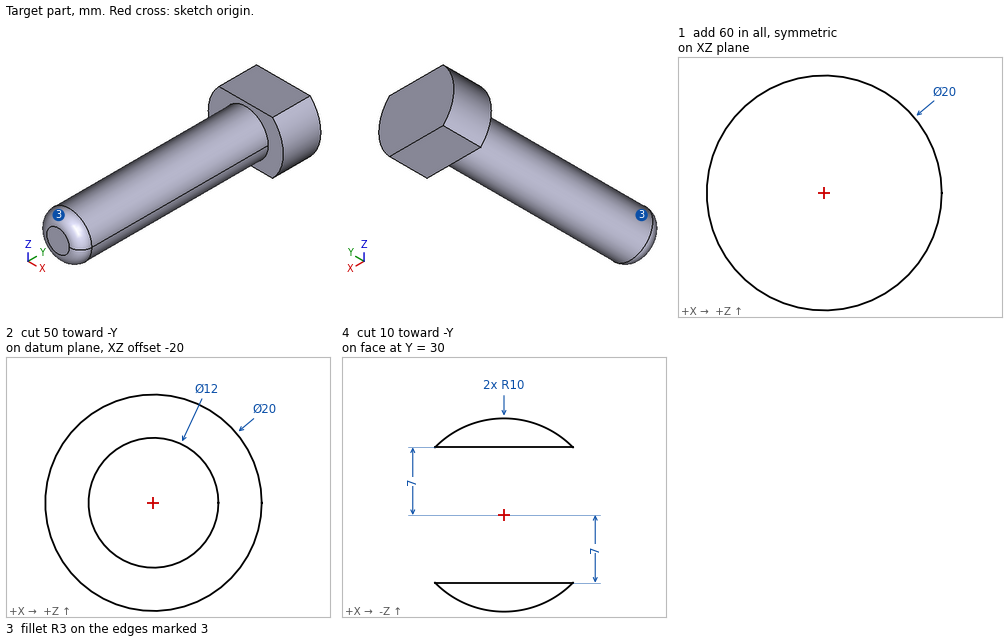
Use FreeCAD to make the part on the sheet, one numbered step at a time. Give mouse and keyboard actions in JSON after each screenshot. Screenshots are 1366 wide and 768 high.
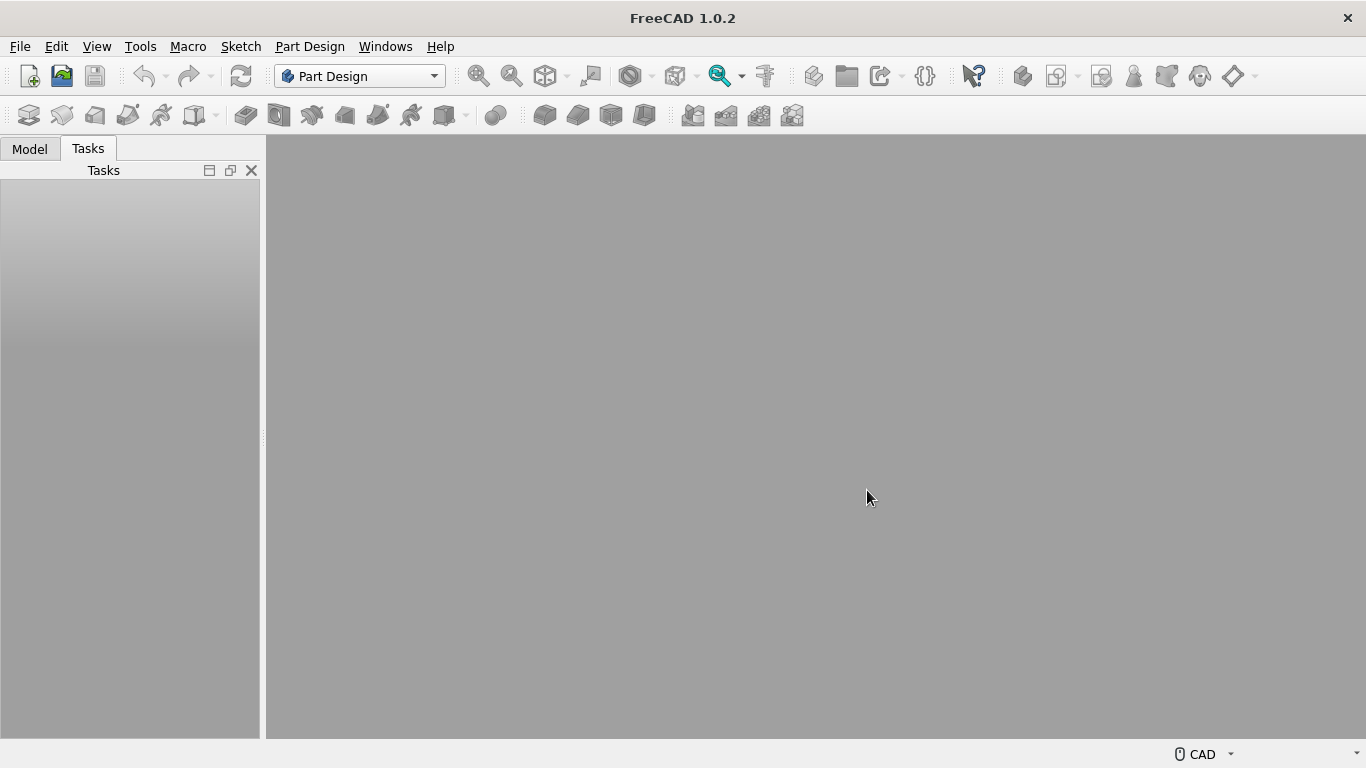
{"action": "left_click", "coordinate": [29, 76]}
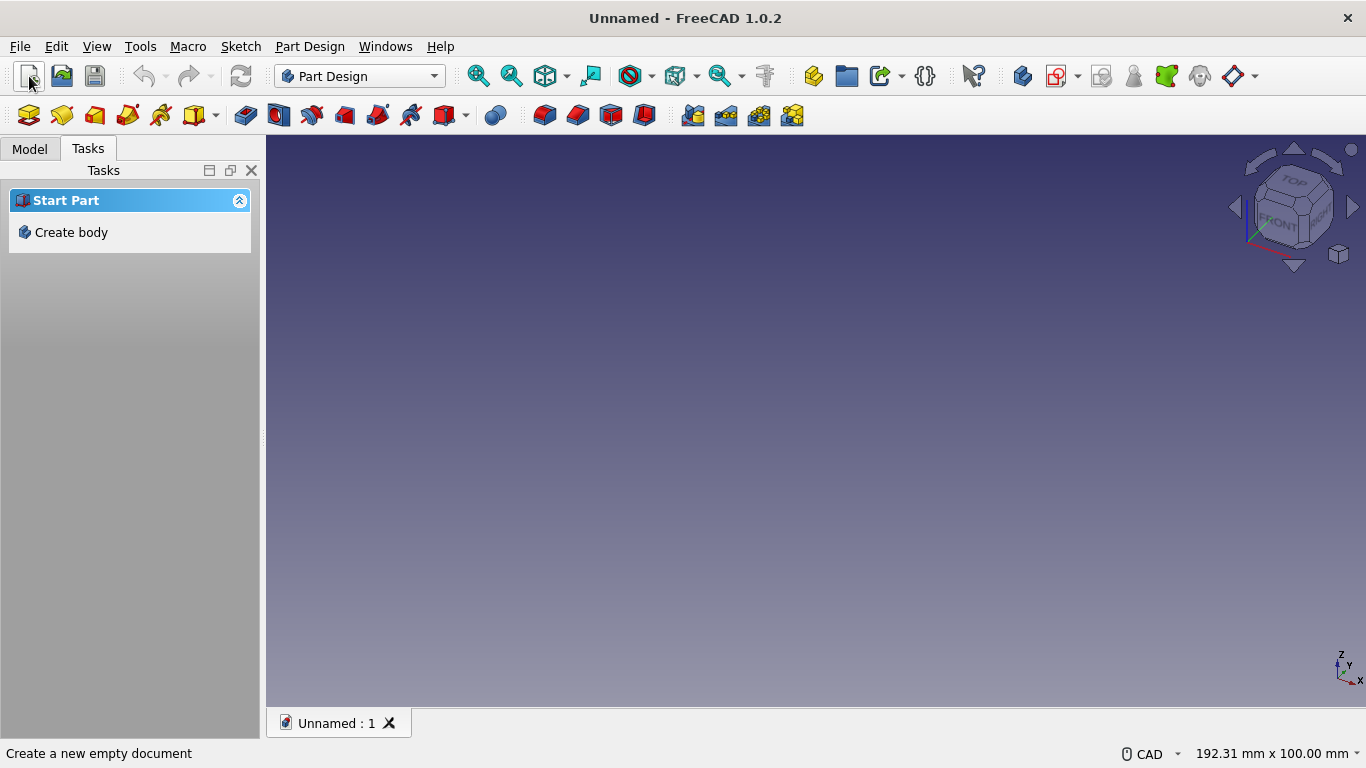
{"action": "left_click", "coordinate": [1056, 76]}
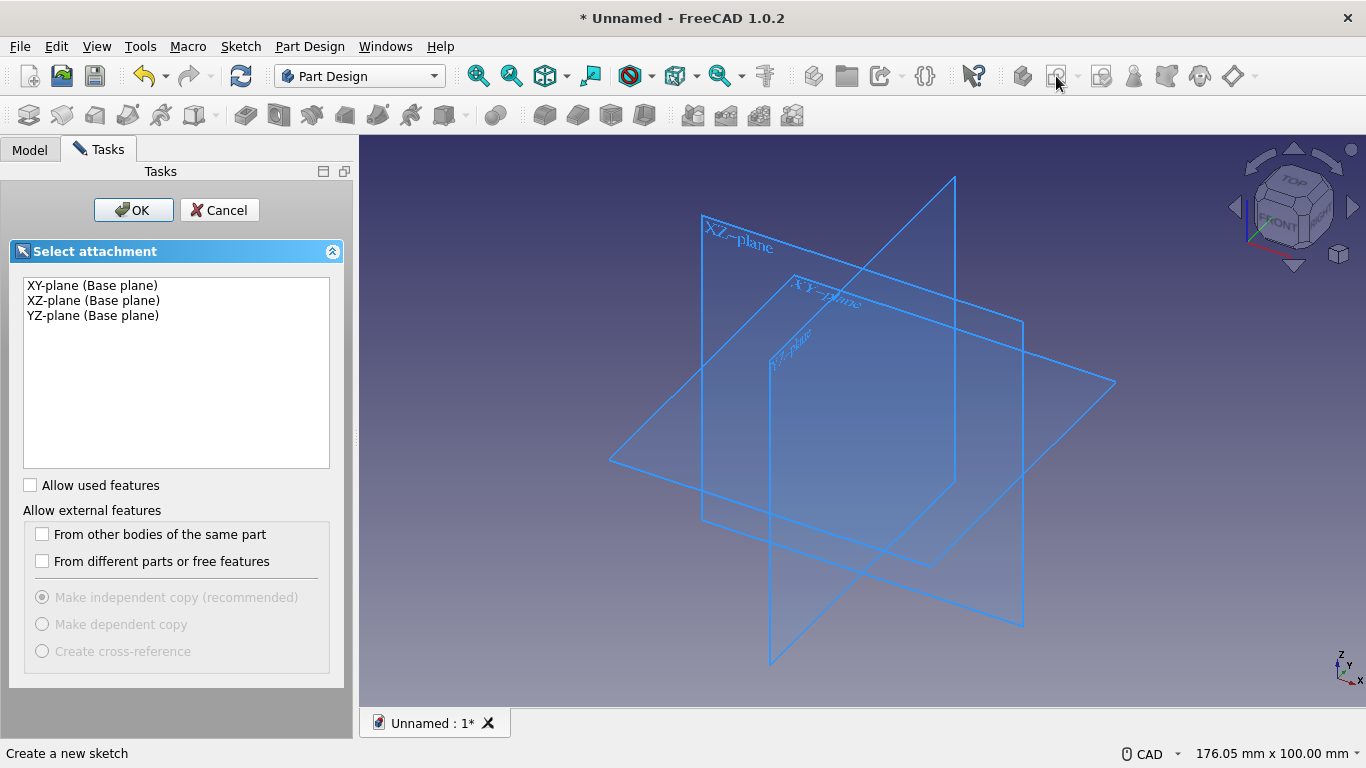
{"action": "left_click", "coordinate": [84, 300]}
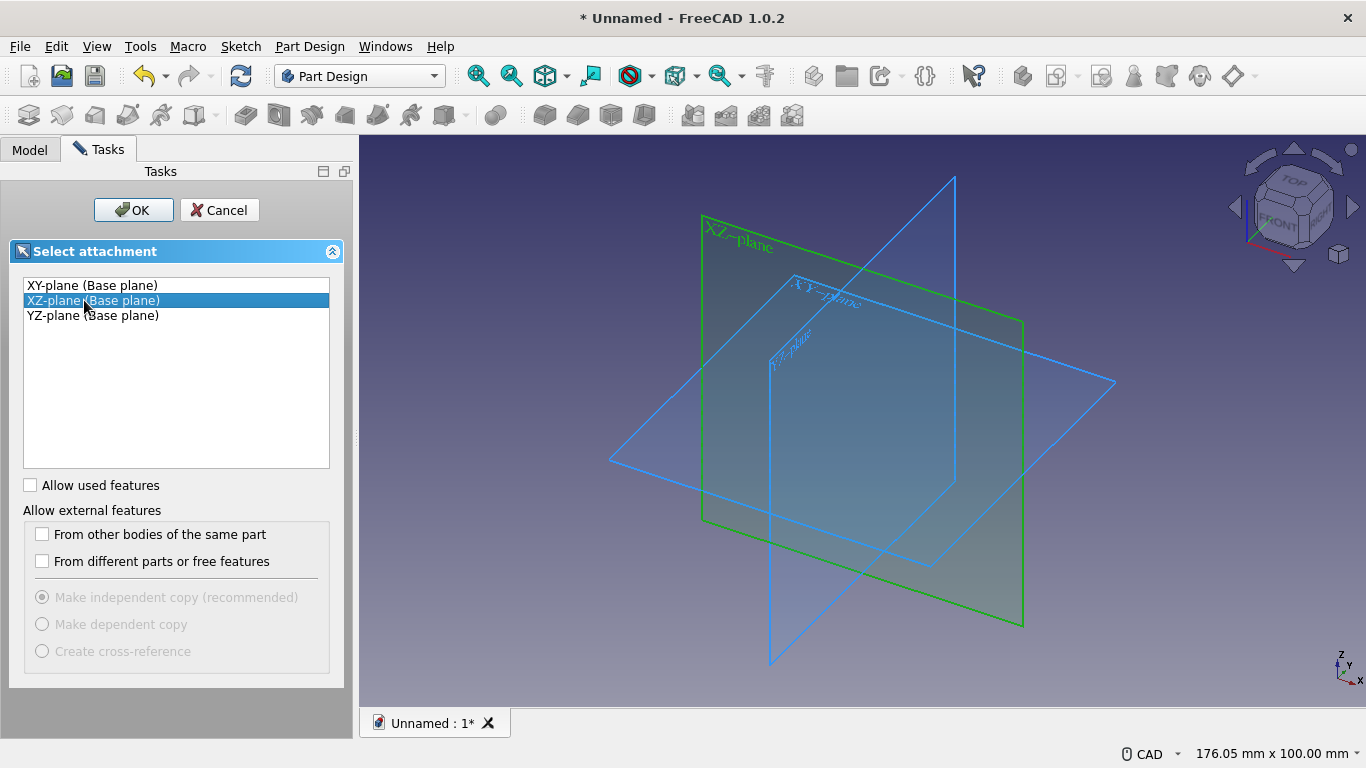
{"action": "left_click", "coordinate": [134, 210]}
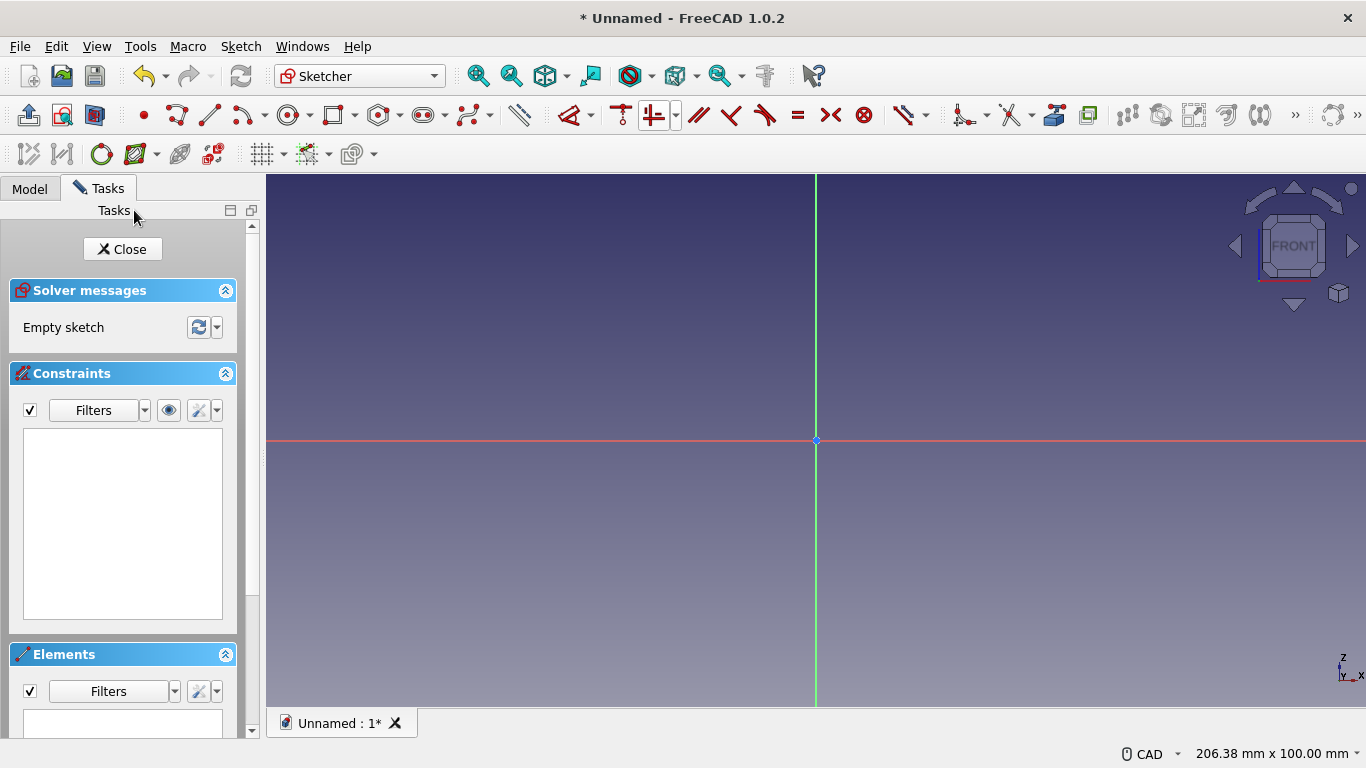
{"action": "scroll", "coordinate": [846, 440], "scroll_direction": "up", "scroll_amount": 6}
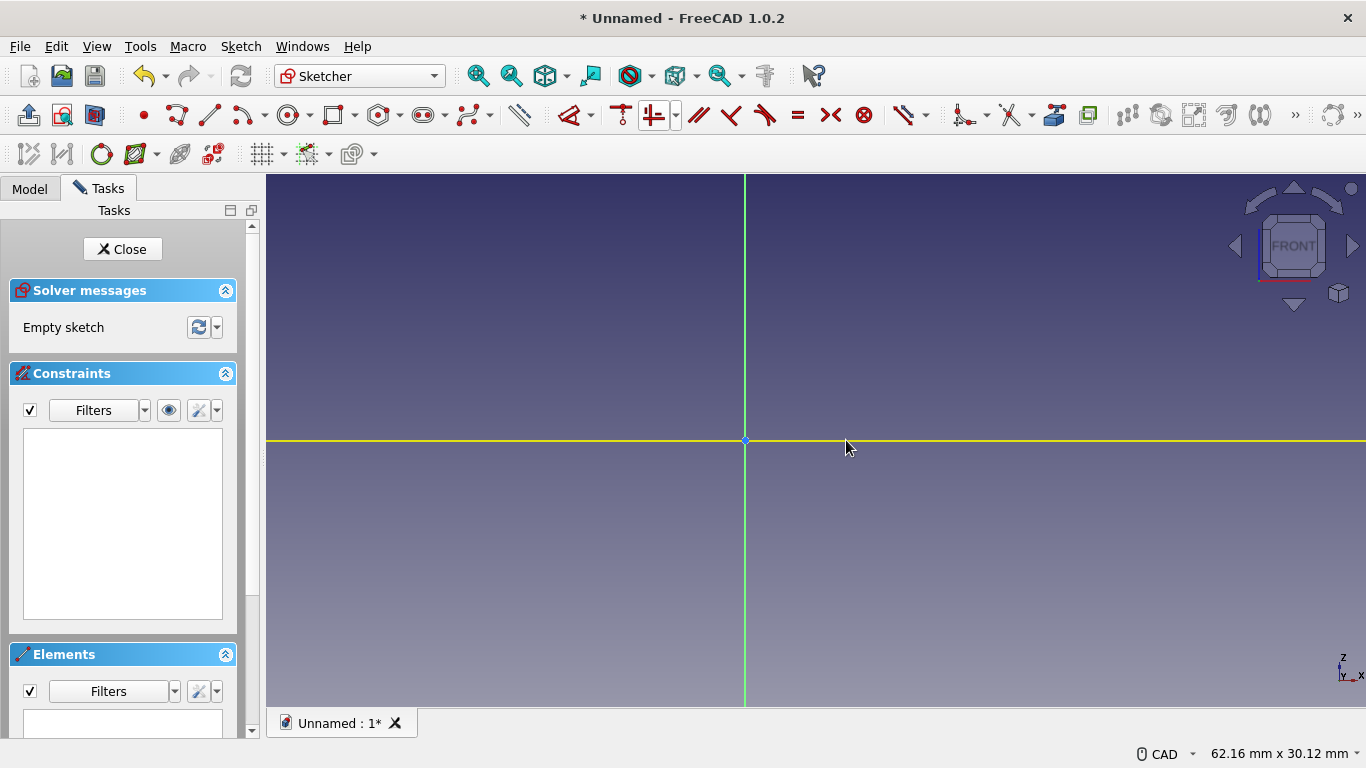
{"action": "left_click", "coordinate": [288, 116]}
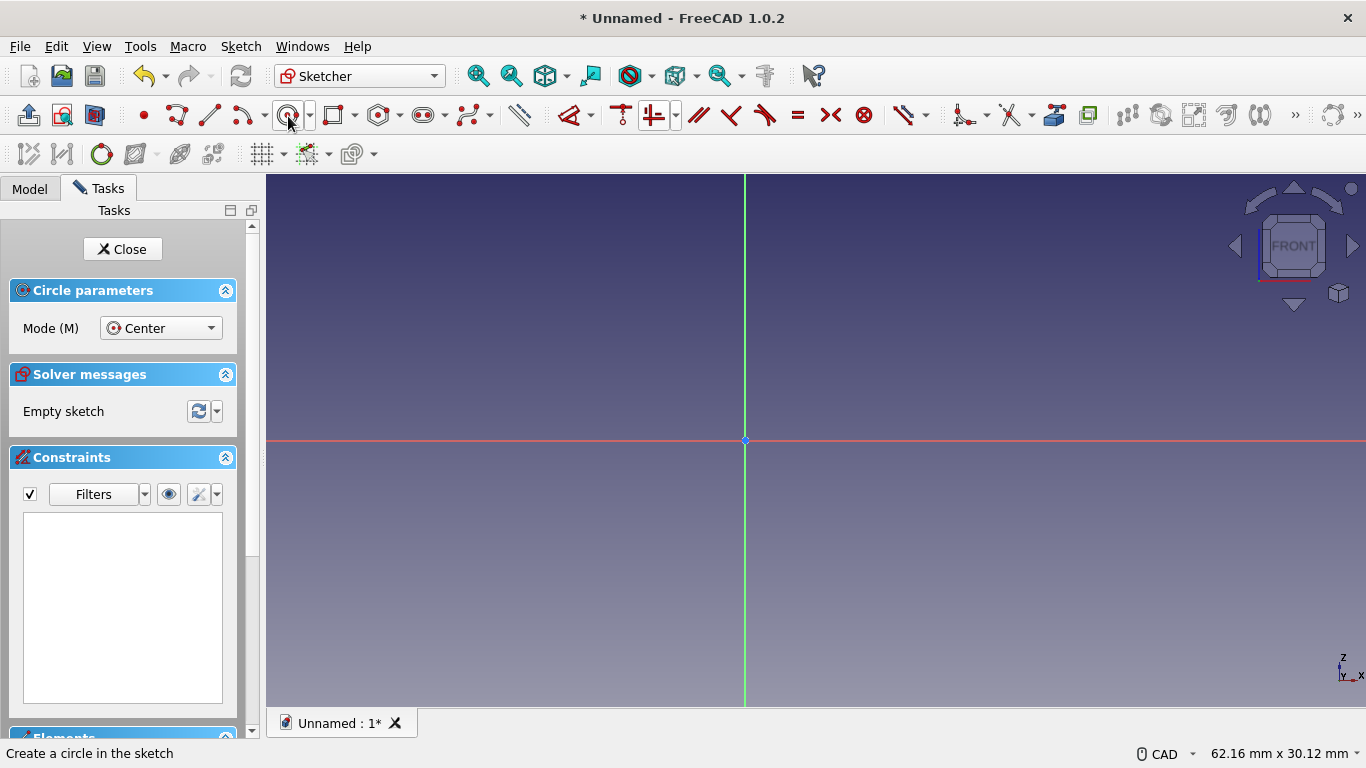
{"action": "left_click", "coordinate": [745, 440]}
{"action": "mouse_move", "coordinate": [870, 315]}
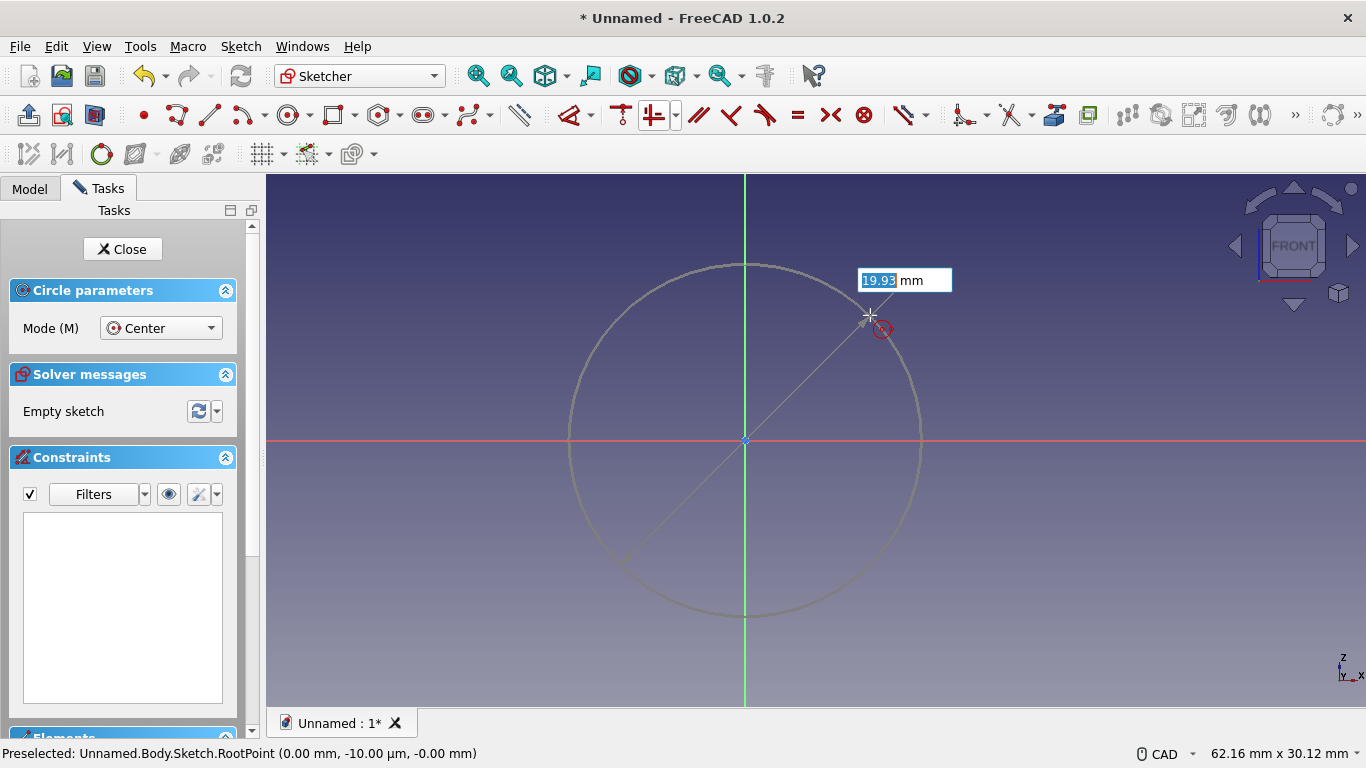
{"action": "type", "text": "20"}
{"action": "key", "text": "Return"}
{"action": "key", "text": "Escape"}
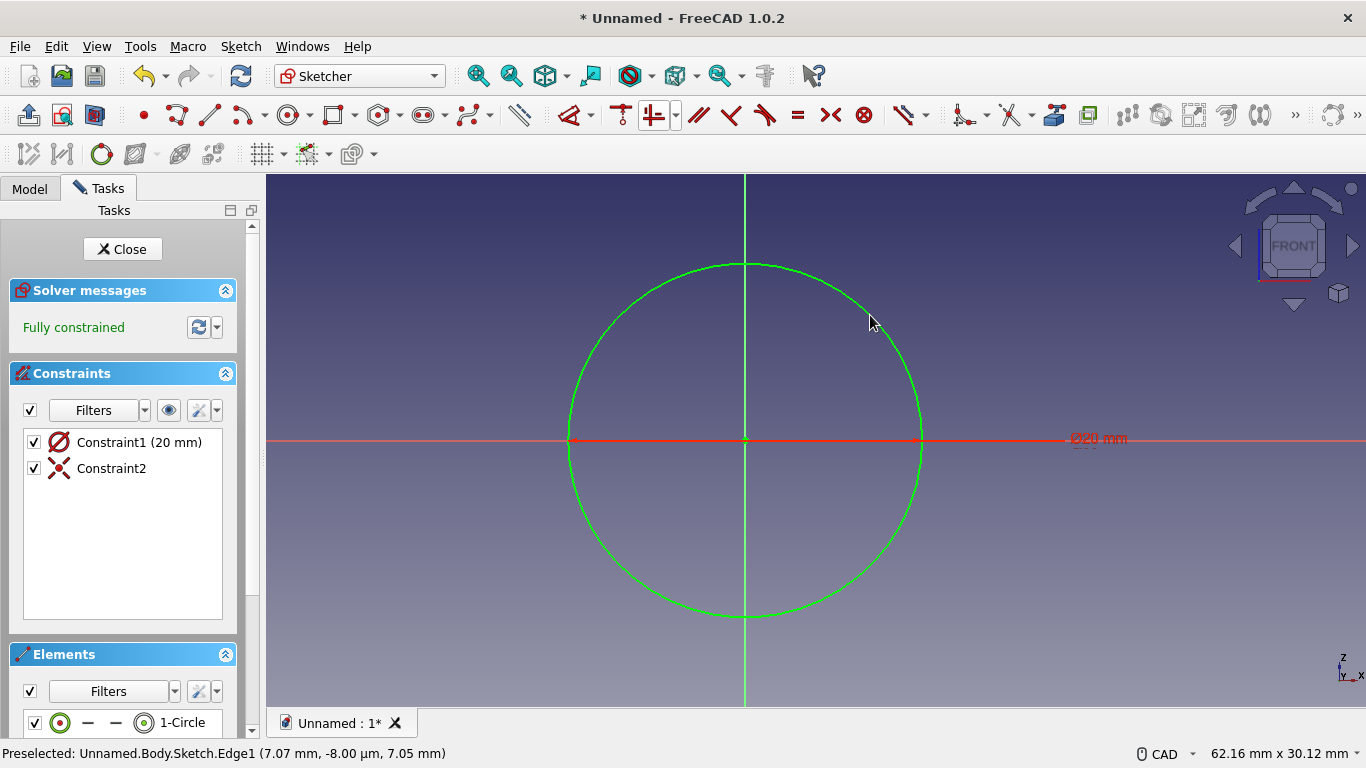
{"action": "left_click", "coordinate": [123, 249]}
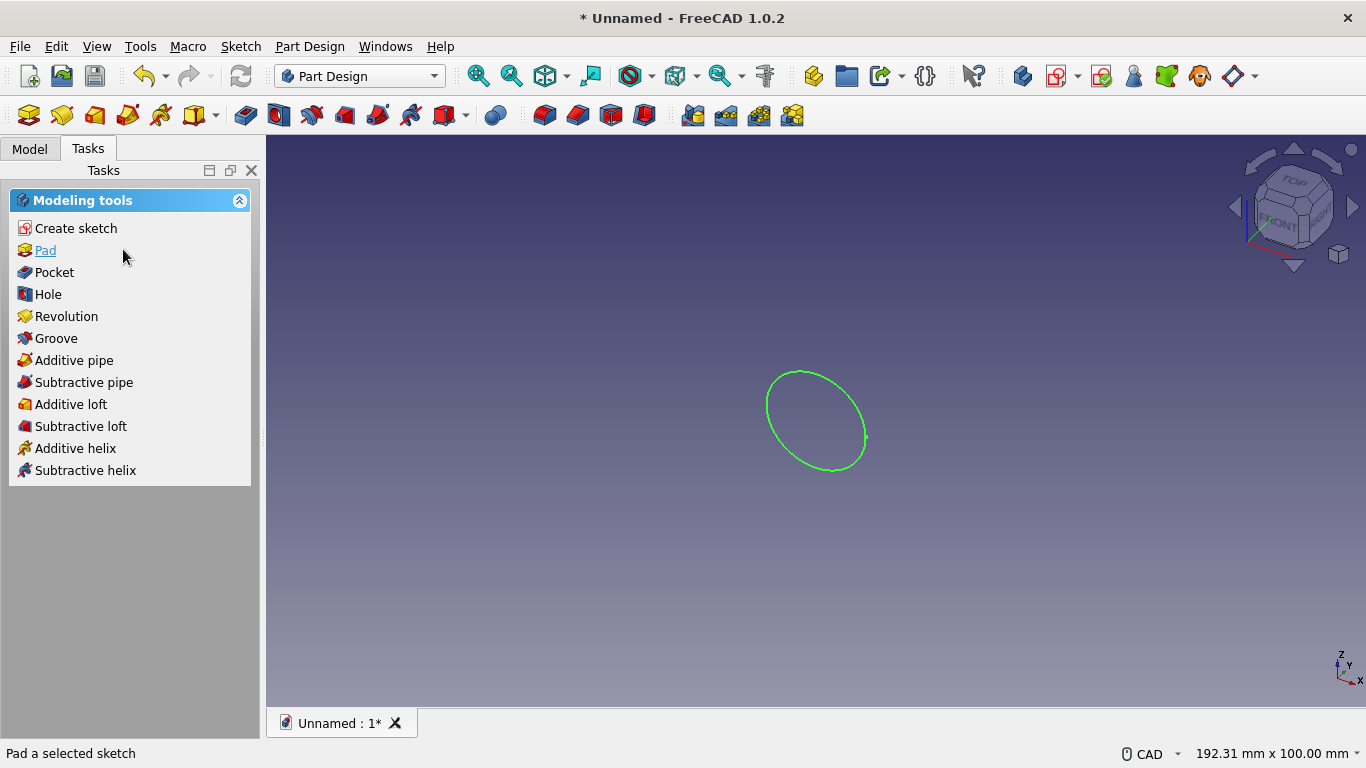
{"action": "left_click", "coordinate": [29, 116]}